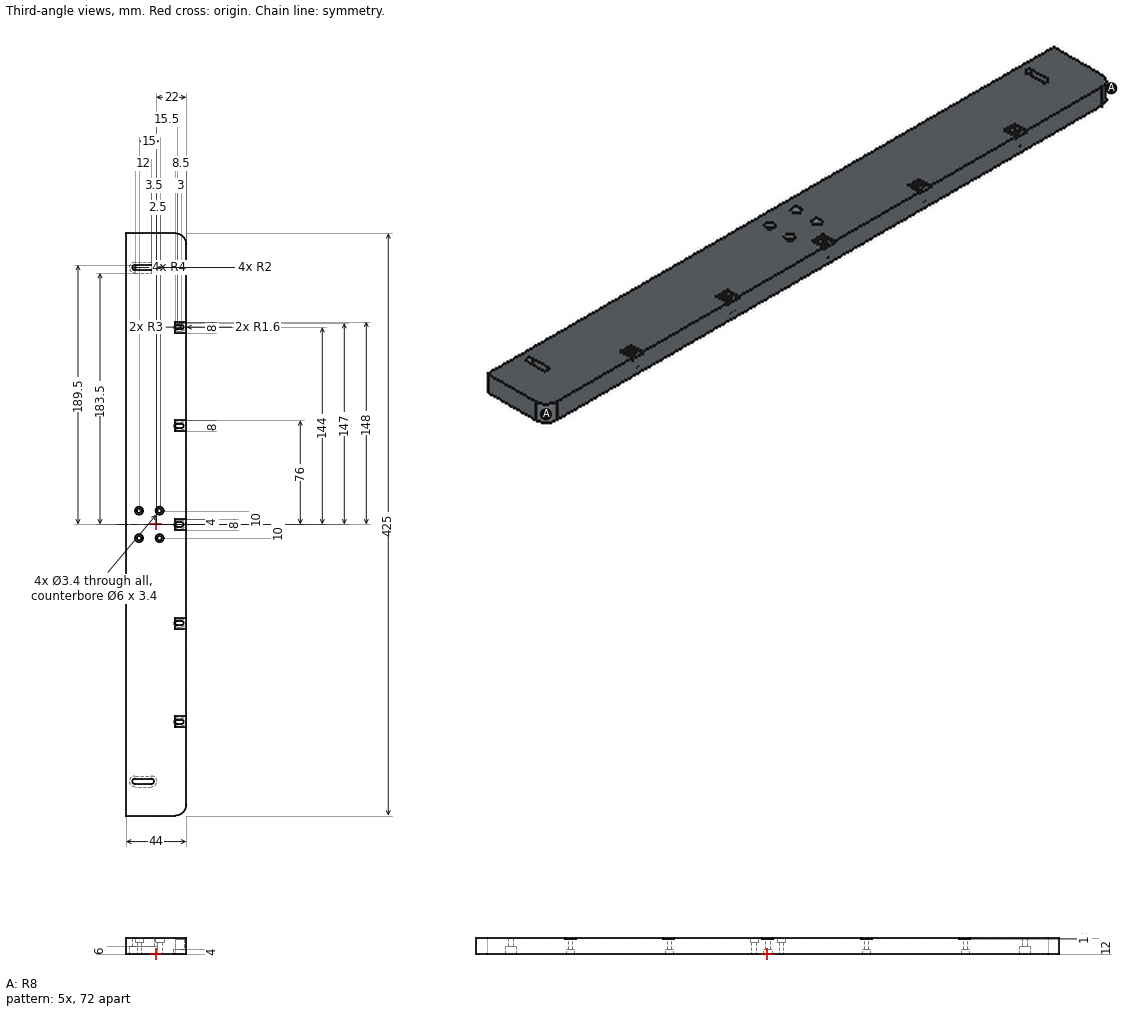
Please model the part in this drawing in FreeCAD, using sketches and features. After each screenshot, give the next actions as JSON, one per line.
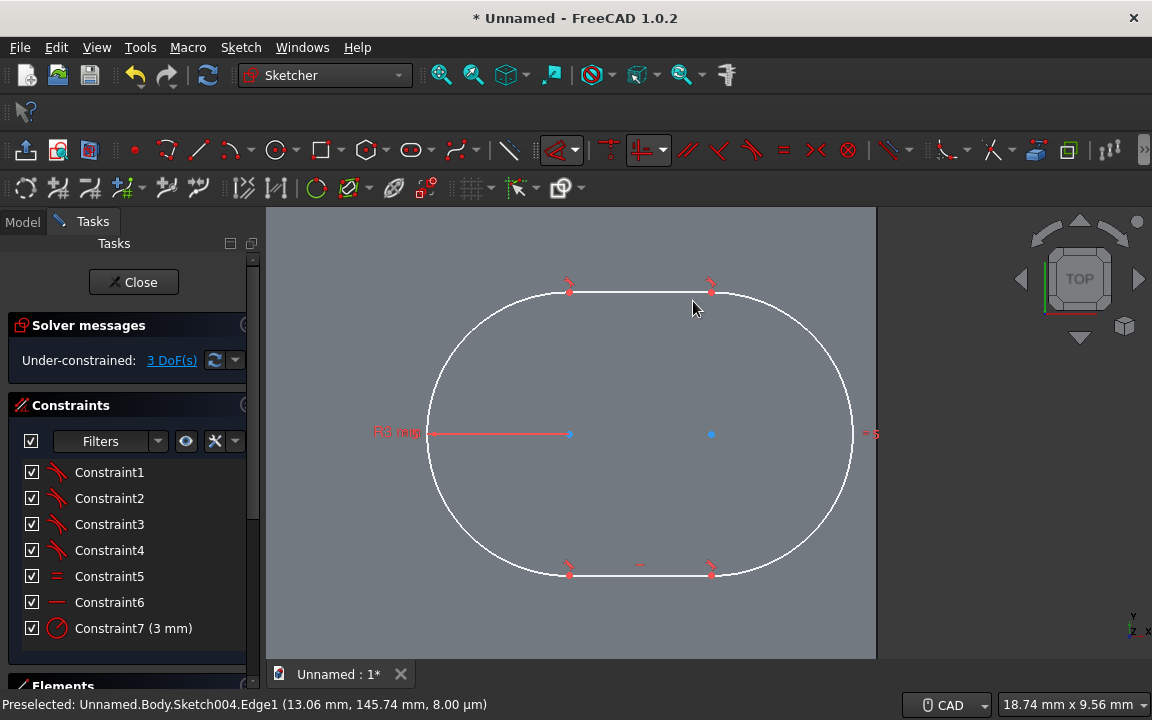
{"action": "left_click", "coordinate": [612, 292]}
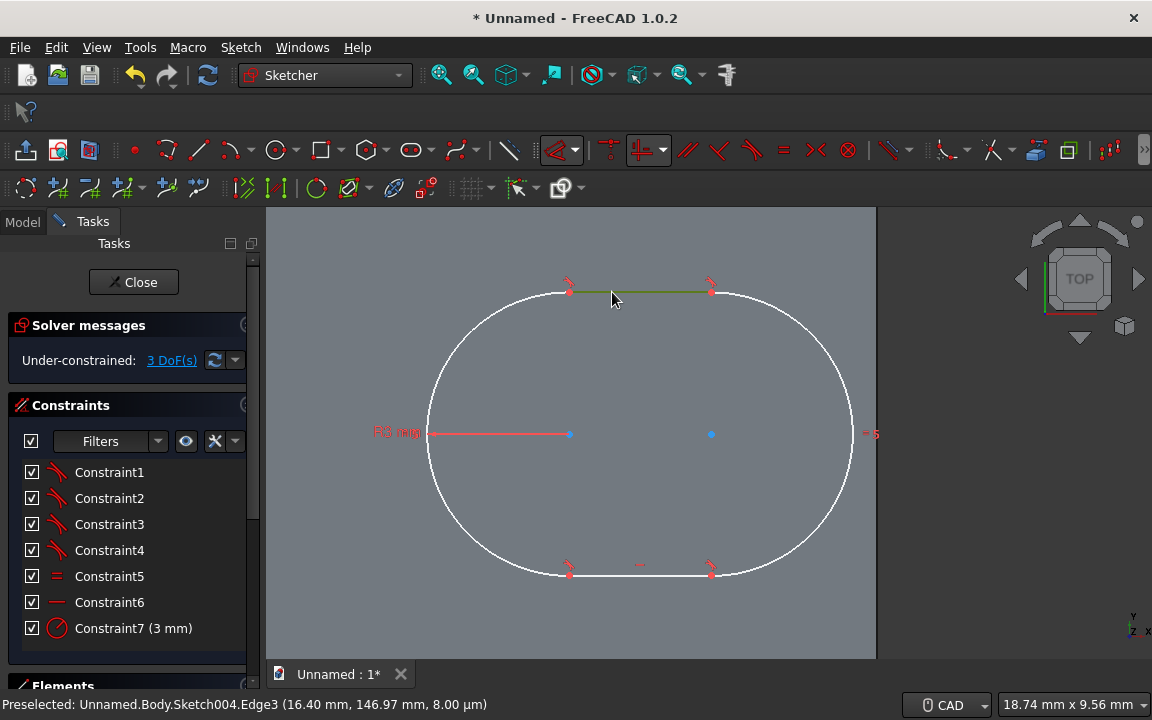
{"action": "left_click", "coordinate": [578, 150]}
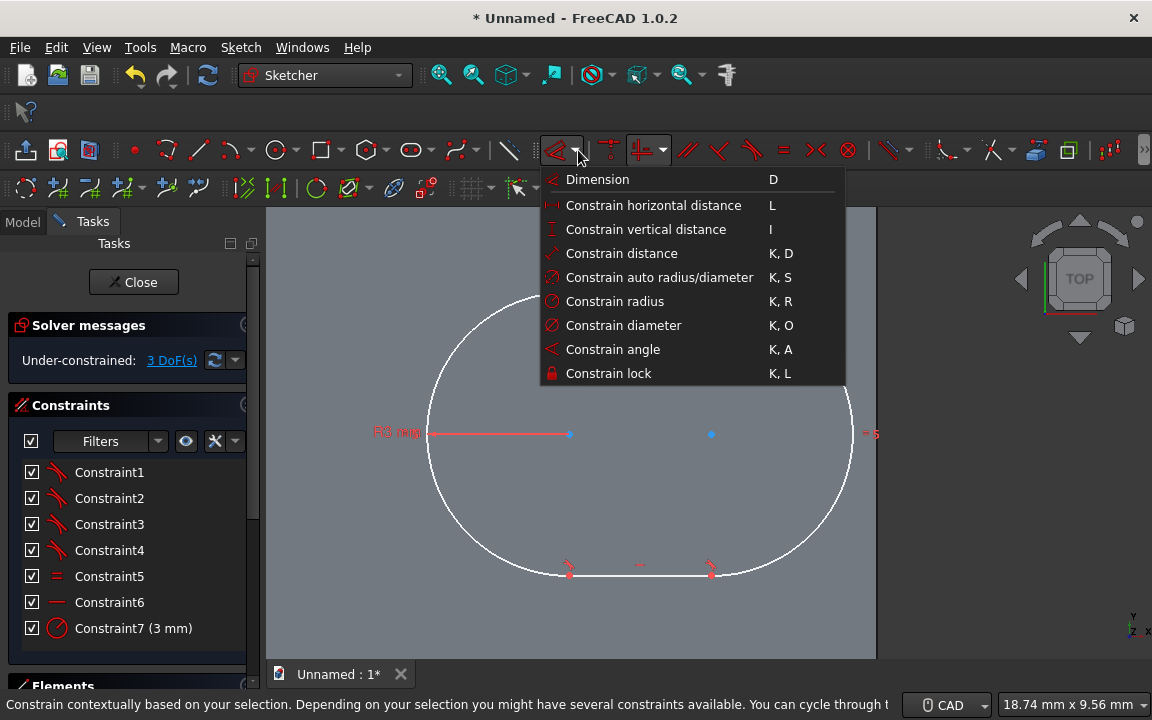
{"action": "left_click", "coordinate": [693, 205]}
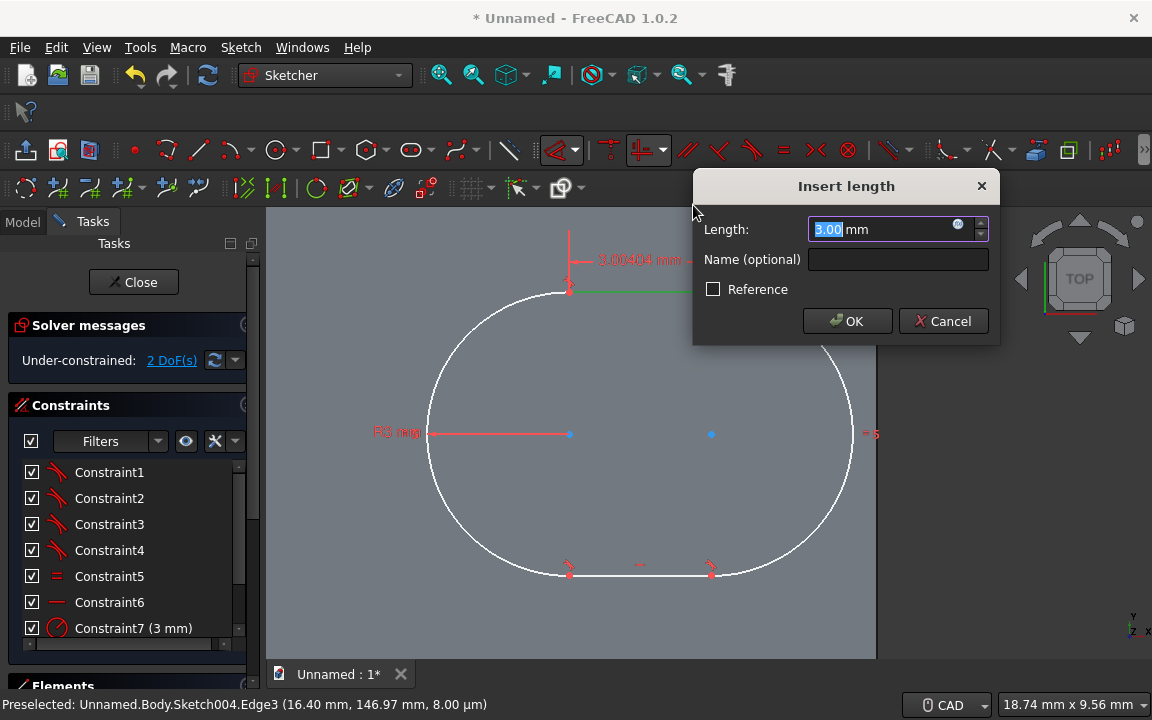
{"action": "type", "text": "3"}
{"action": "key", "text": "Return"}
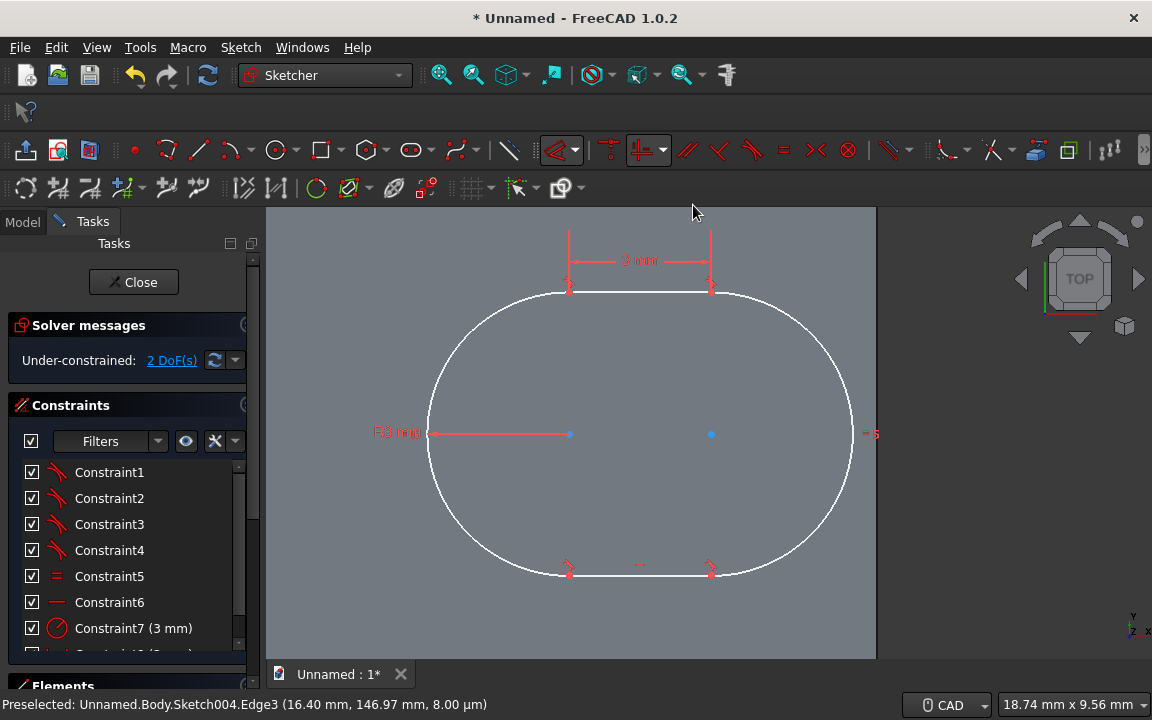
{"action": "left_click", "coordinate": [569, 292]}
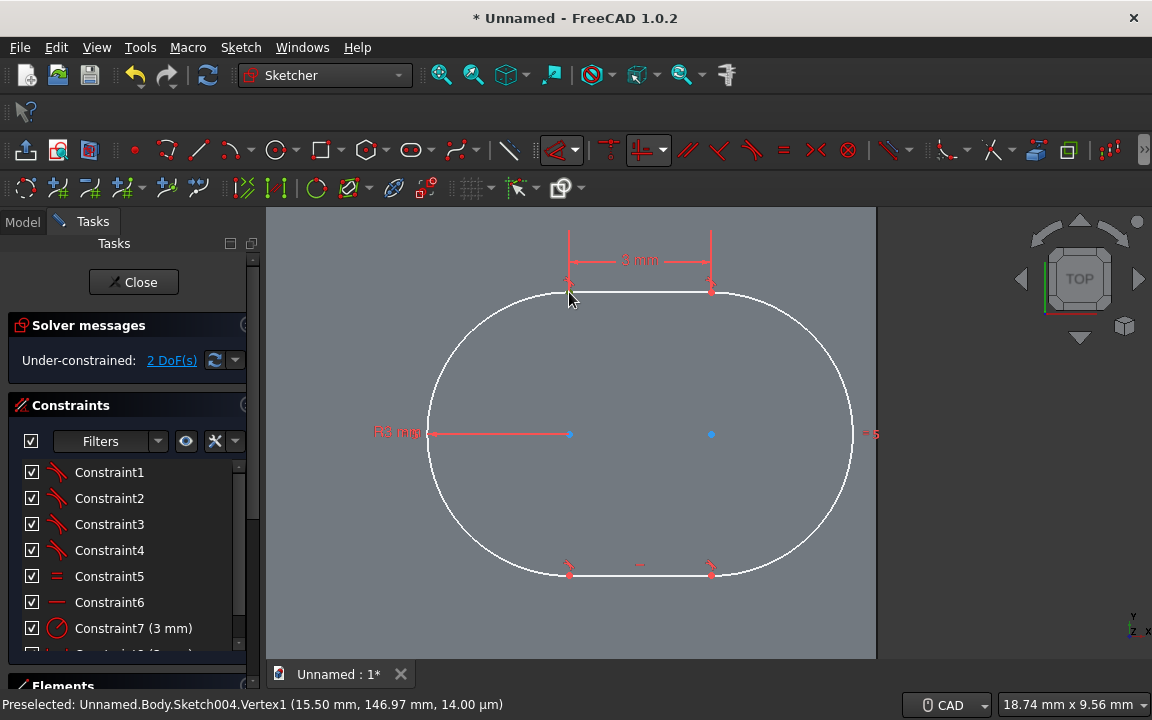
{"action": "left_click", "coordinate": [578, 150]}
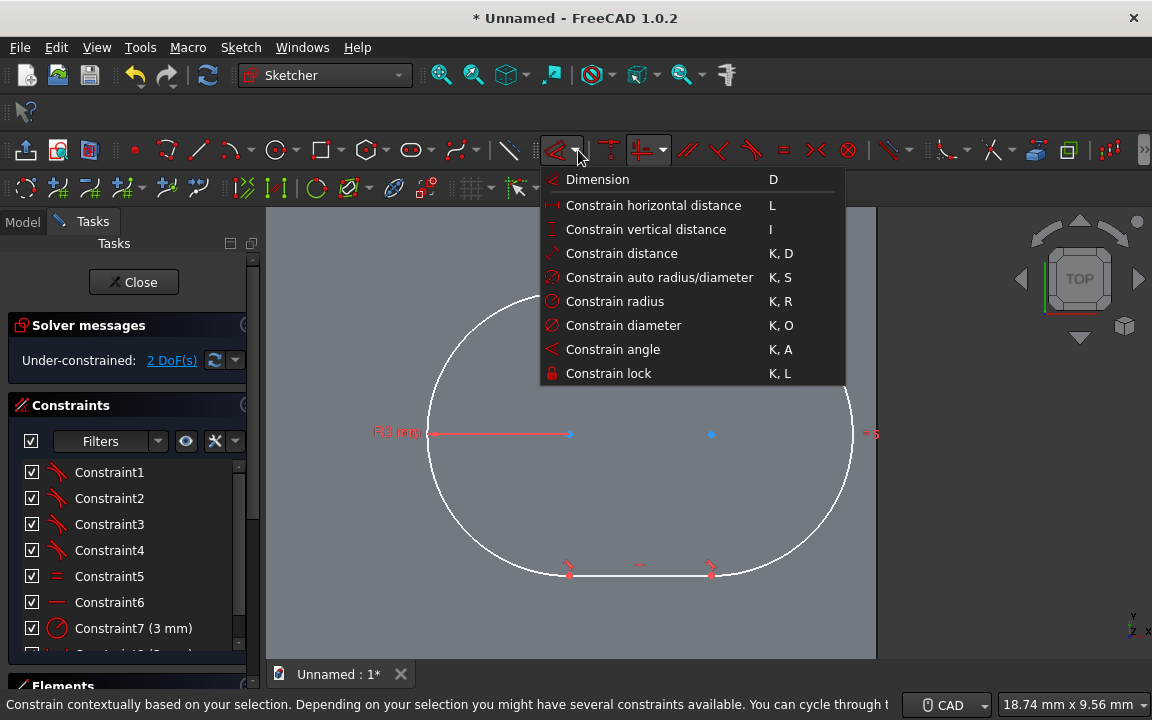
{"action": "left_click", "coordinate": [693, 229]}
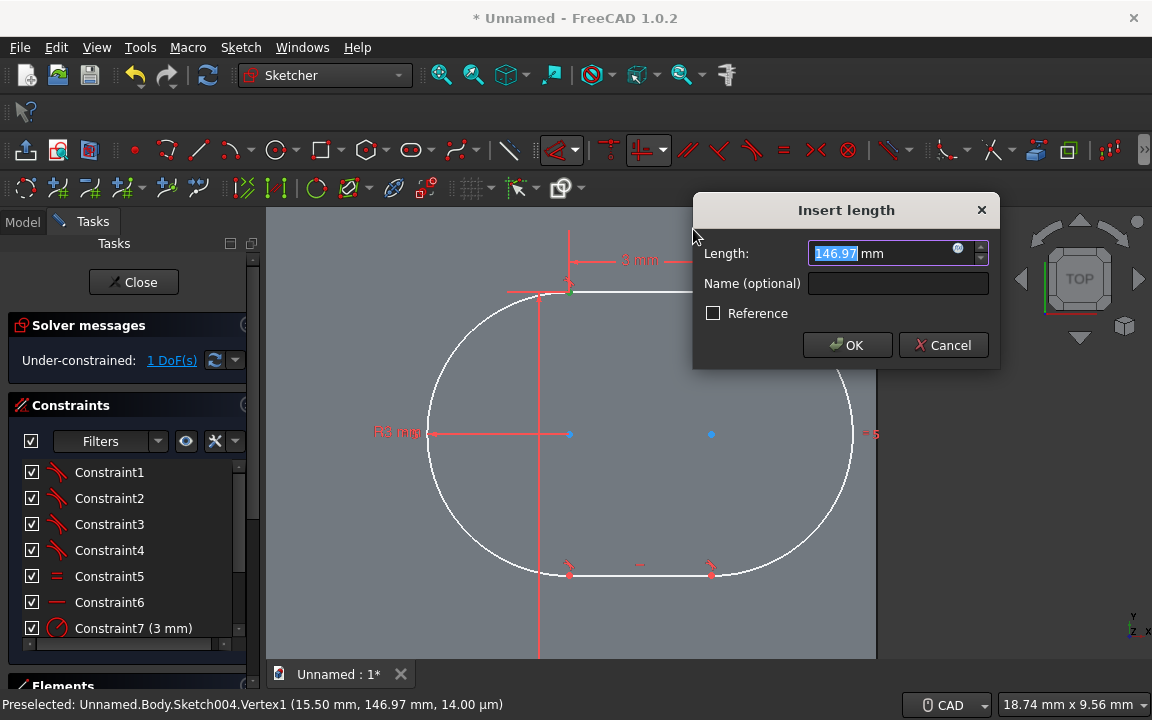
{"action": "type", "text": "147"}
{"action": "key", "text": "Return"}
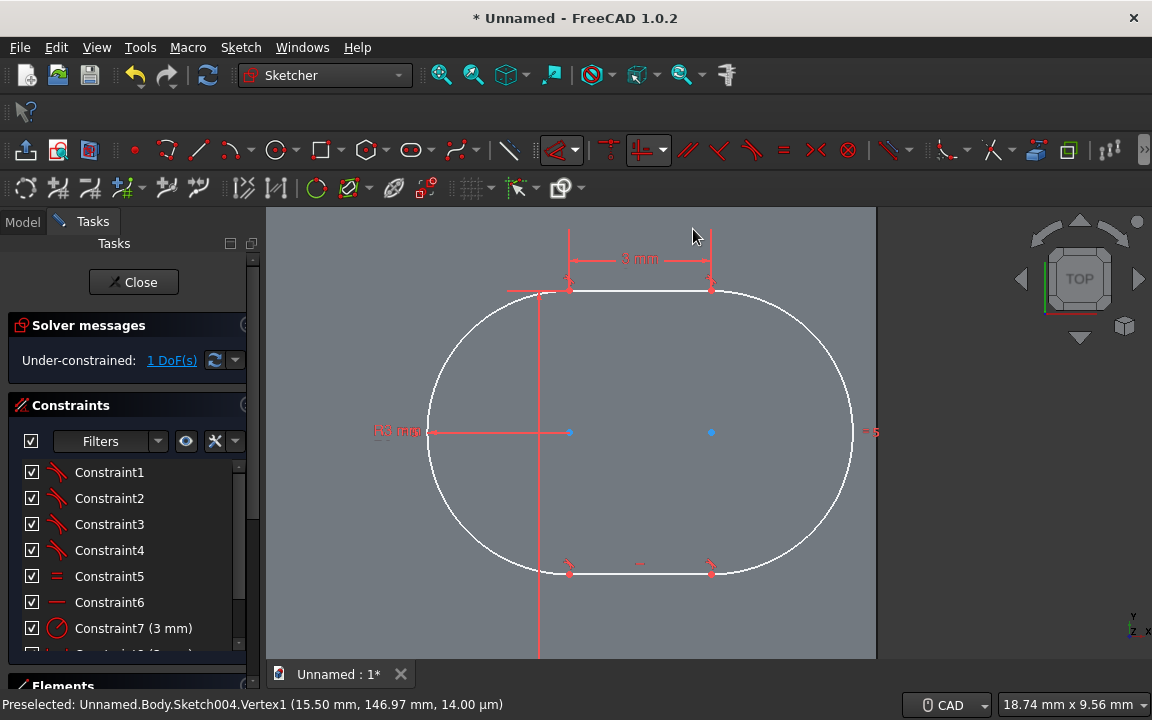
{"action": "left_click", "coordinate": [569, 291]}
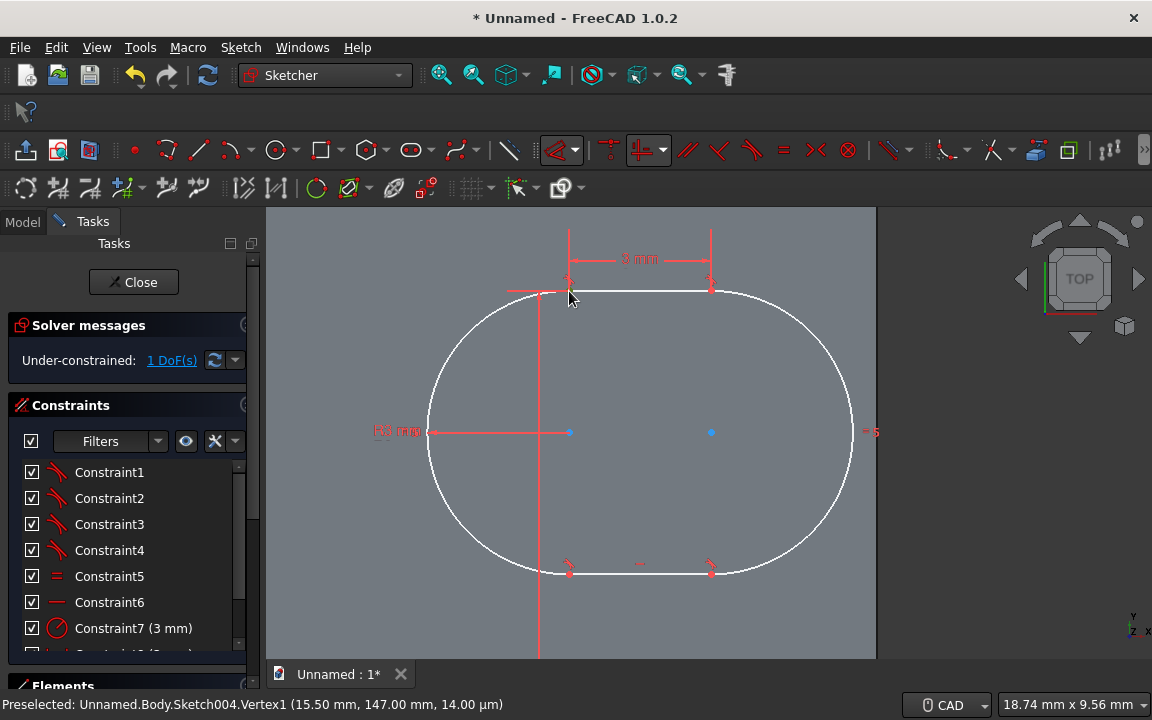
{"action": "key", "text": "l"}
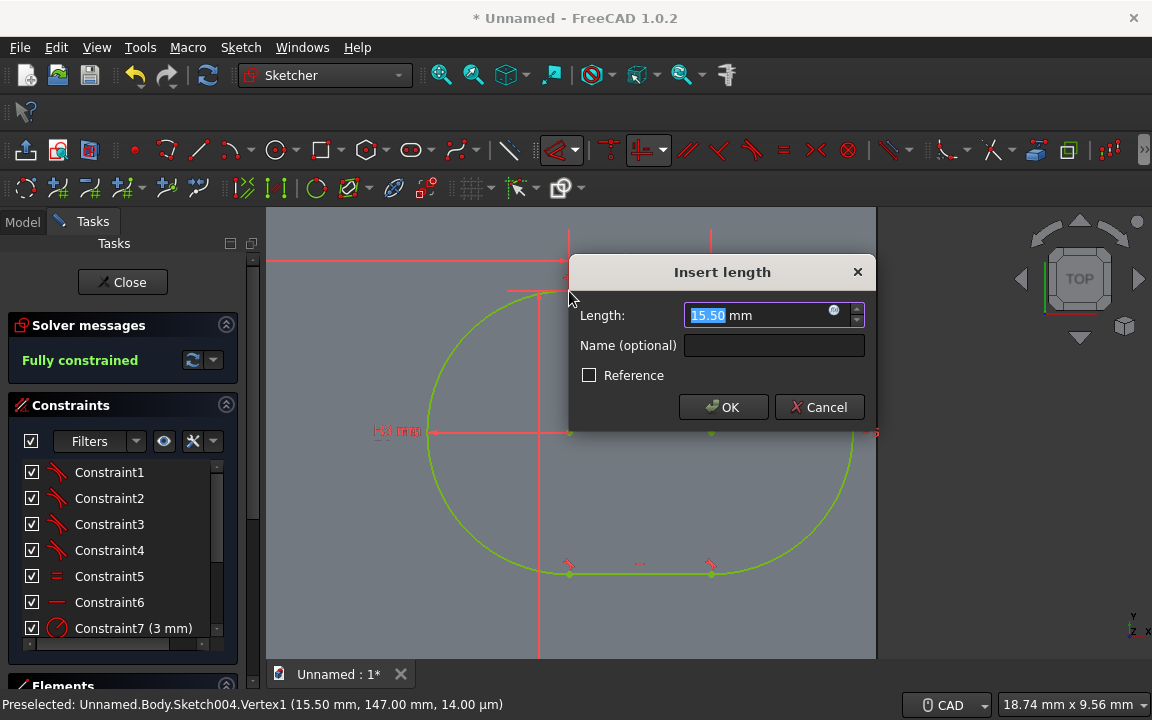
{"action": "type", "text": "15.5"}
{"action": "key", "text": "Return"}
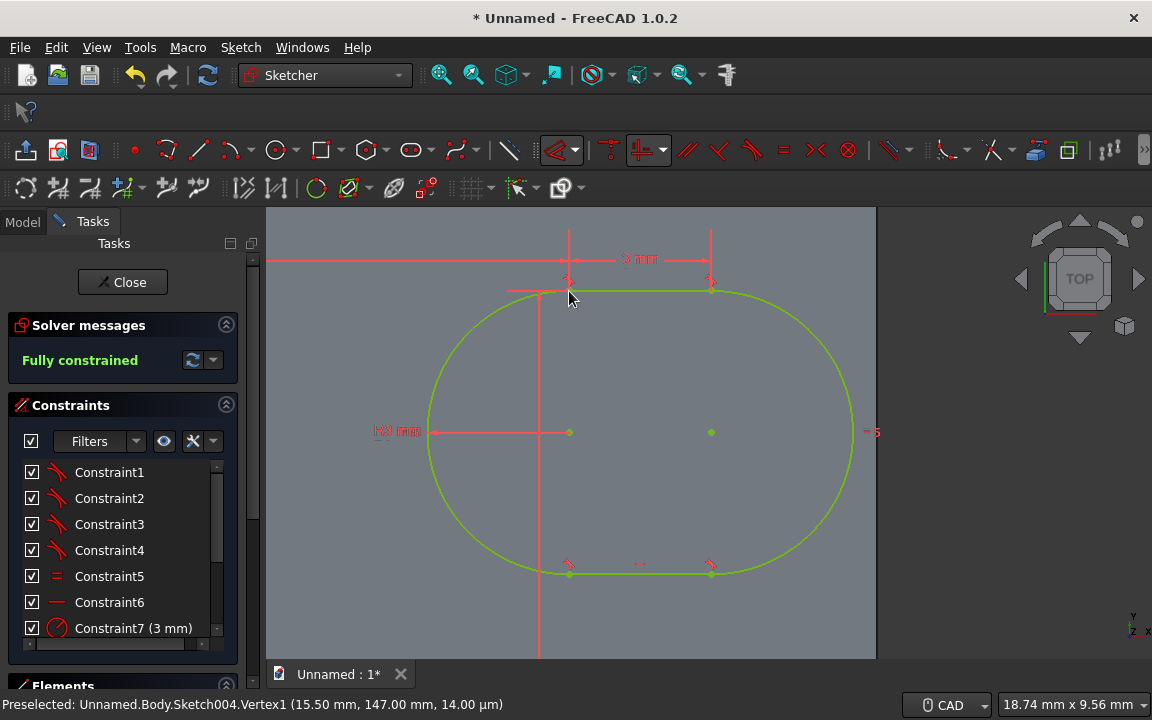
{"action": "left_click", "coordinate": [123, 282]}